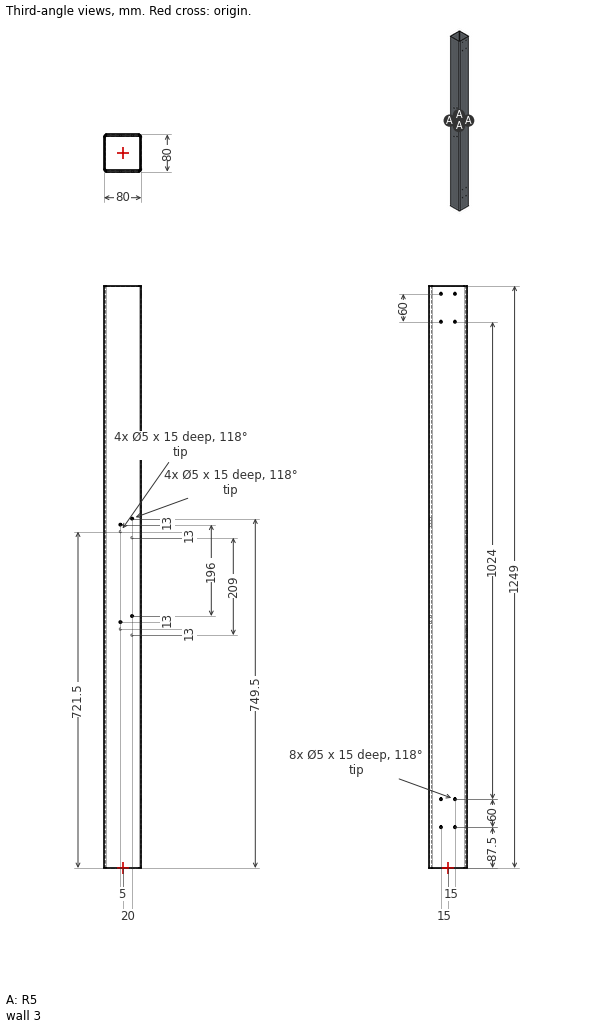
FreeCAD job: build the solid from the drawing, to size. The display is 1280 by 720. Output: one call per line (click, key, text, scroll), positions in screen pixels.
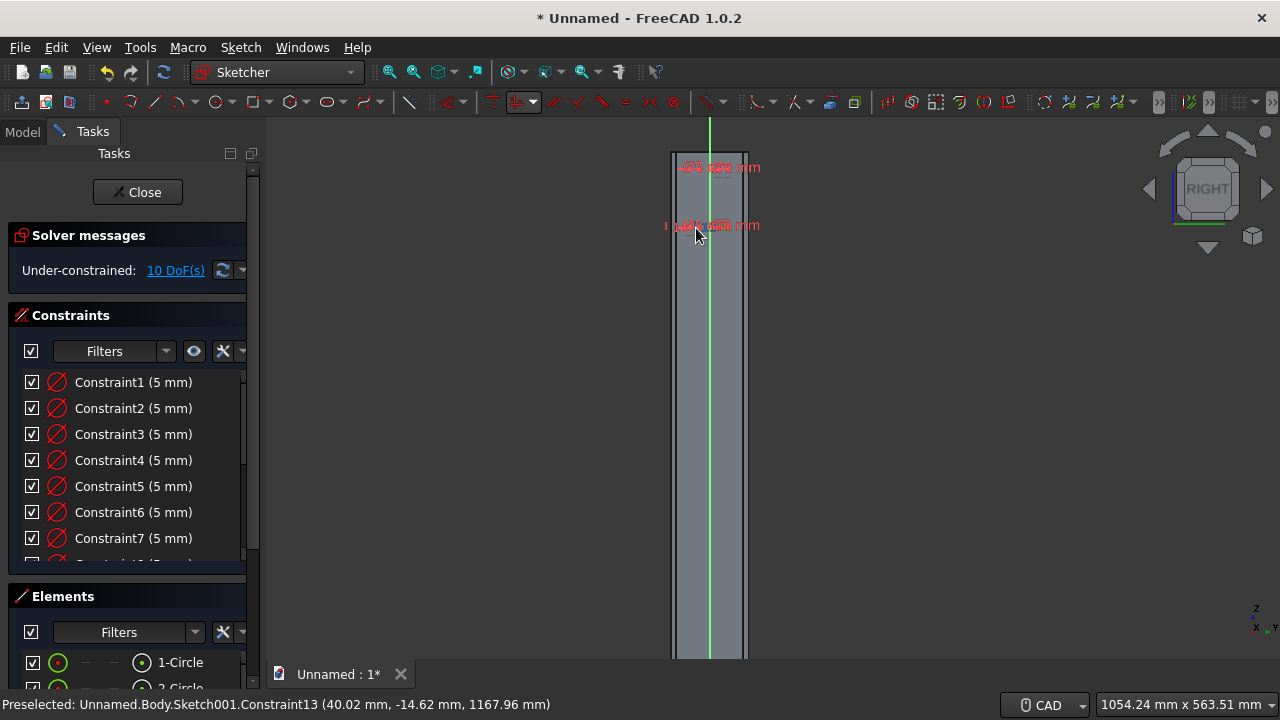
scroll(695, 228, up, 4)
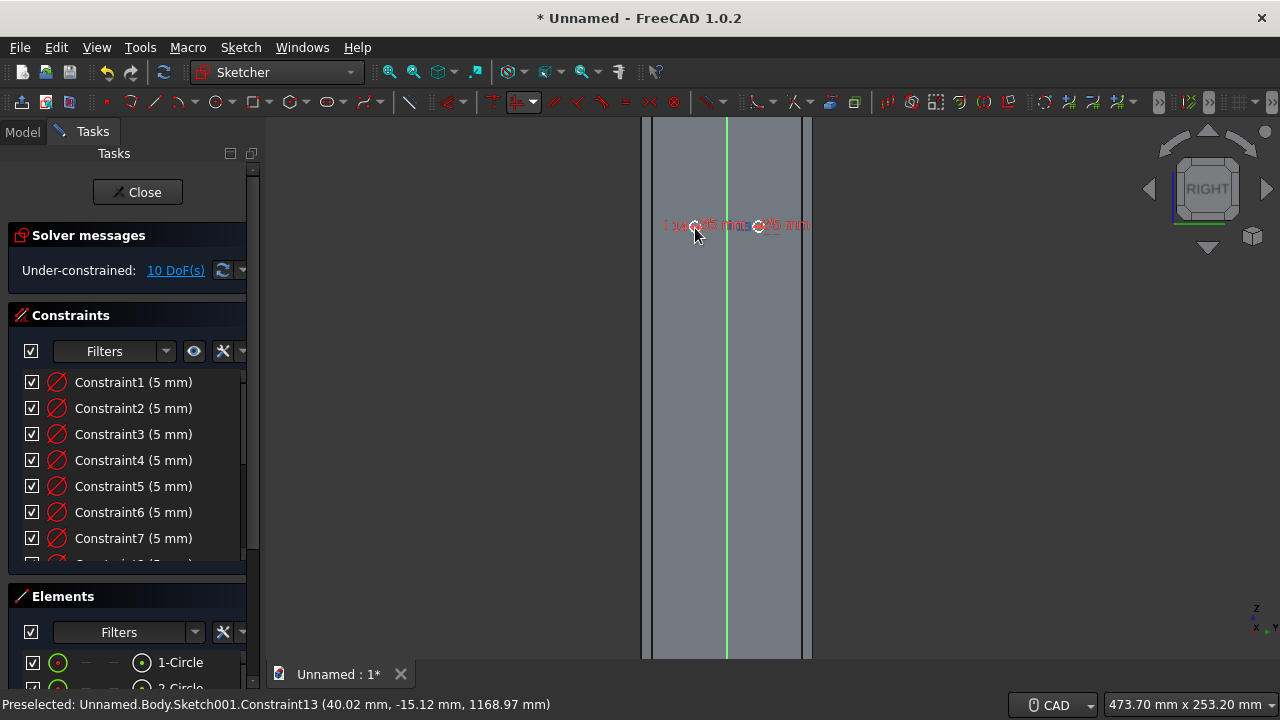
click(695, 227)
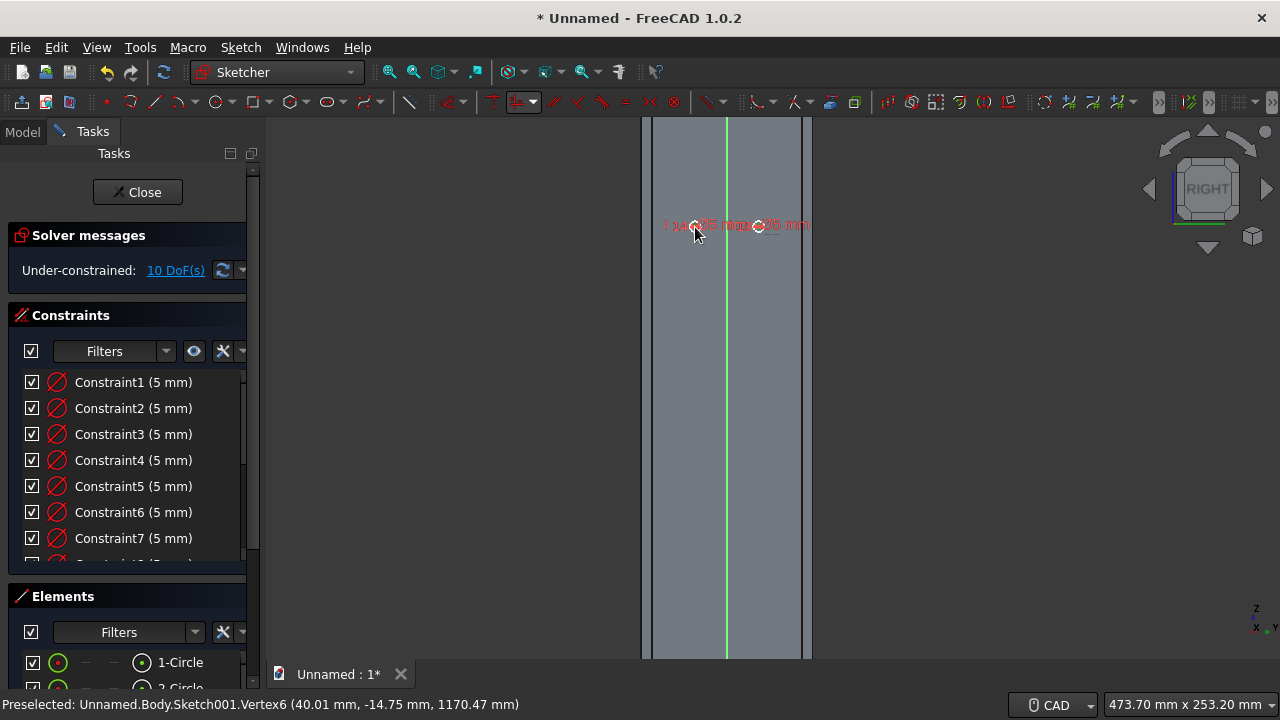
key(h)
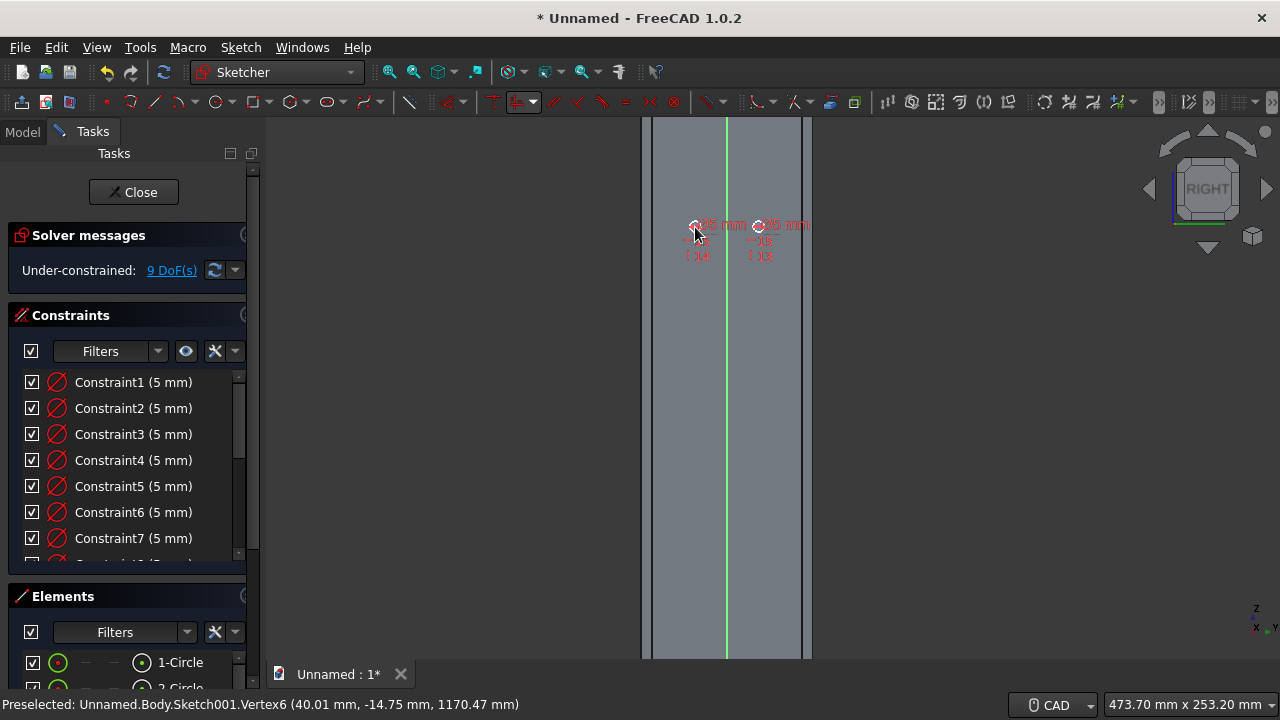
scroll(701, 228, down, 10)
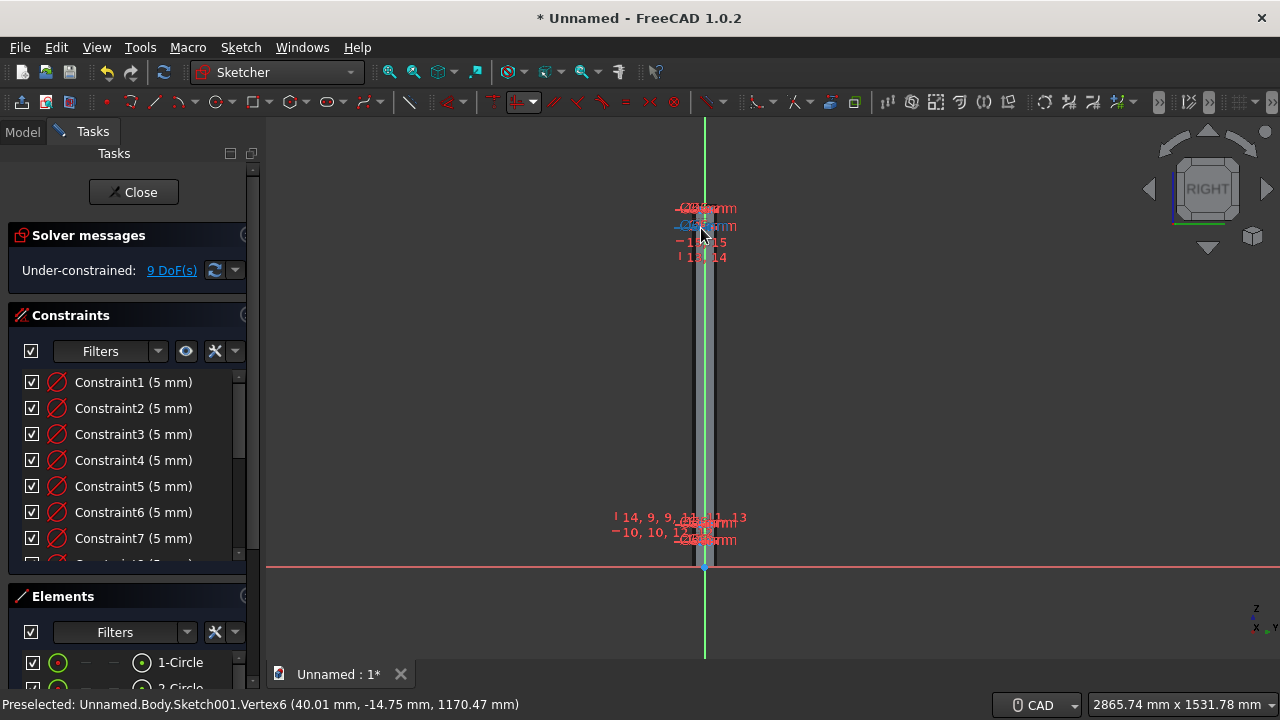
scroll(701, 228, up, 2)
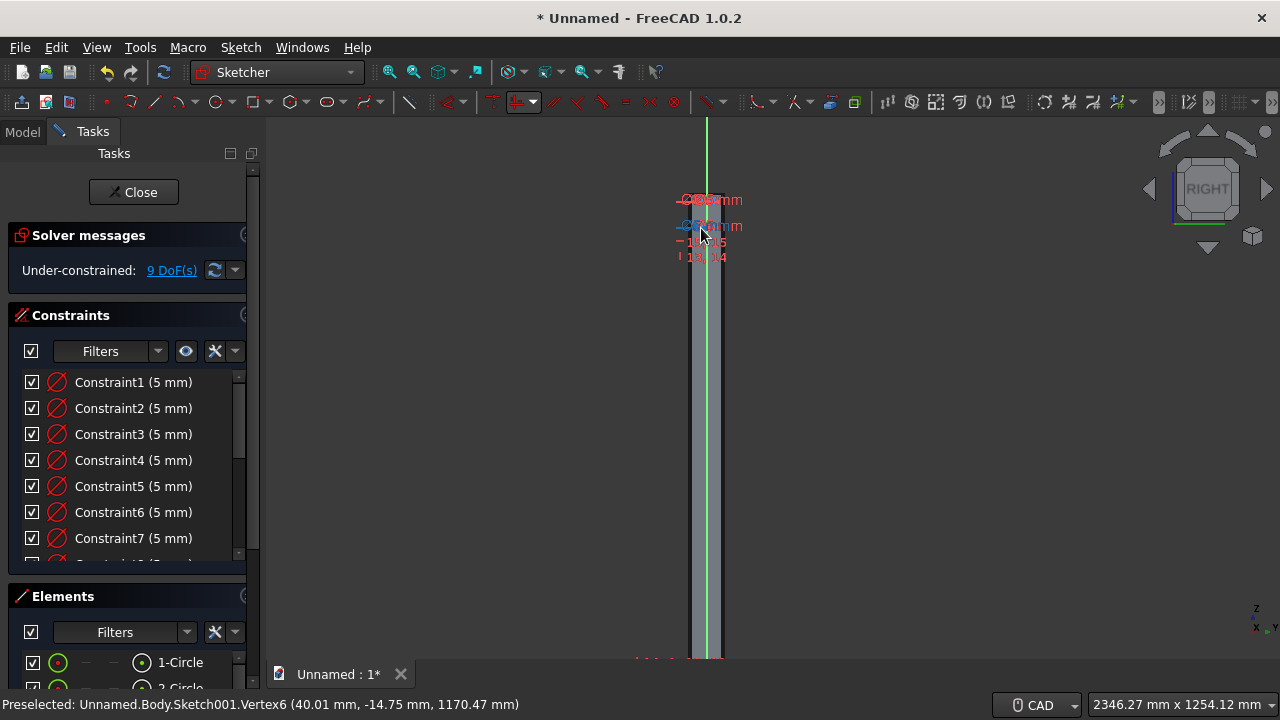
click(700, 228)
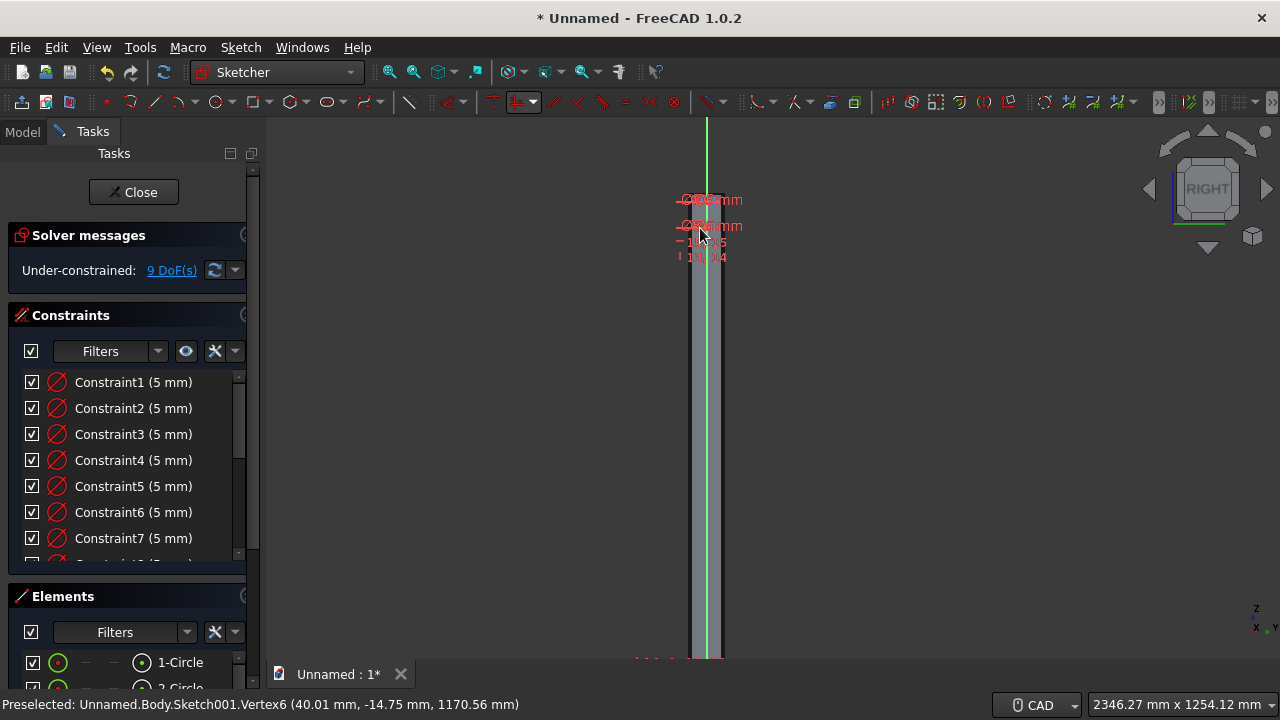
click(700, 202)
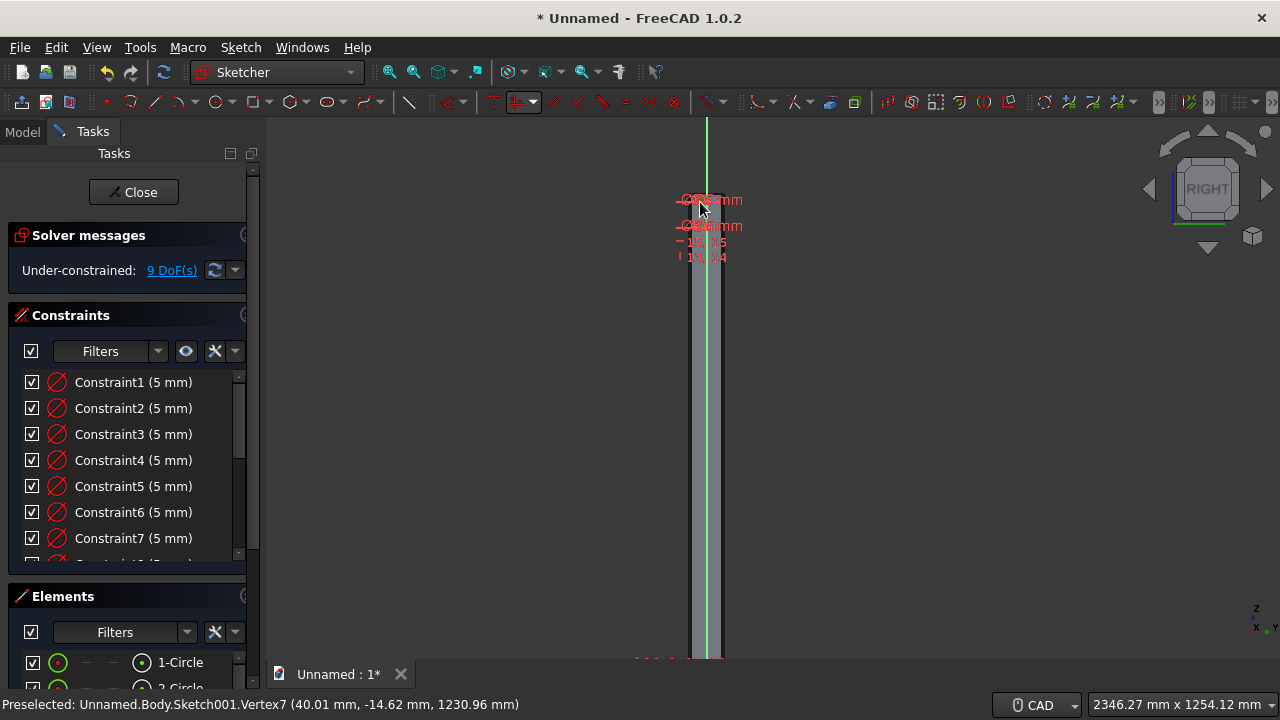
key(v)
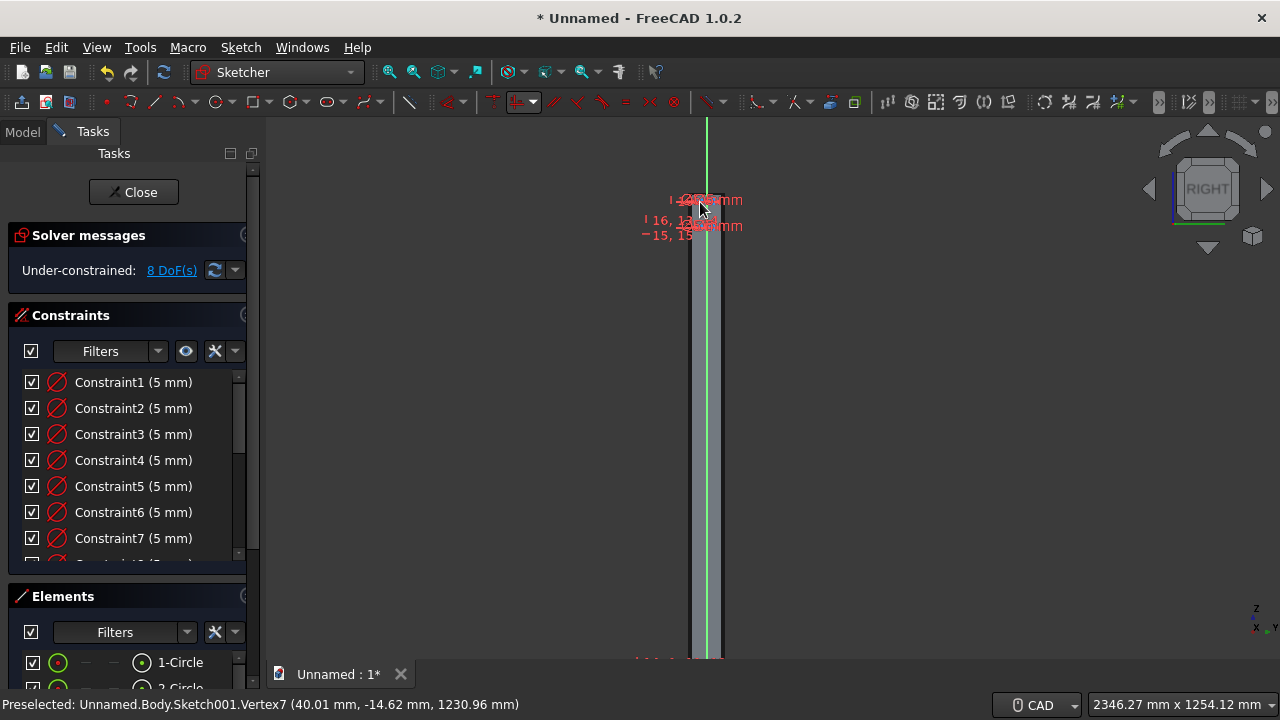
click(713, 228)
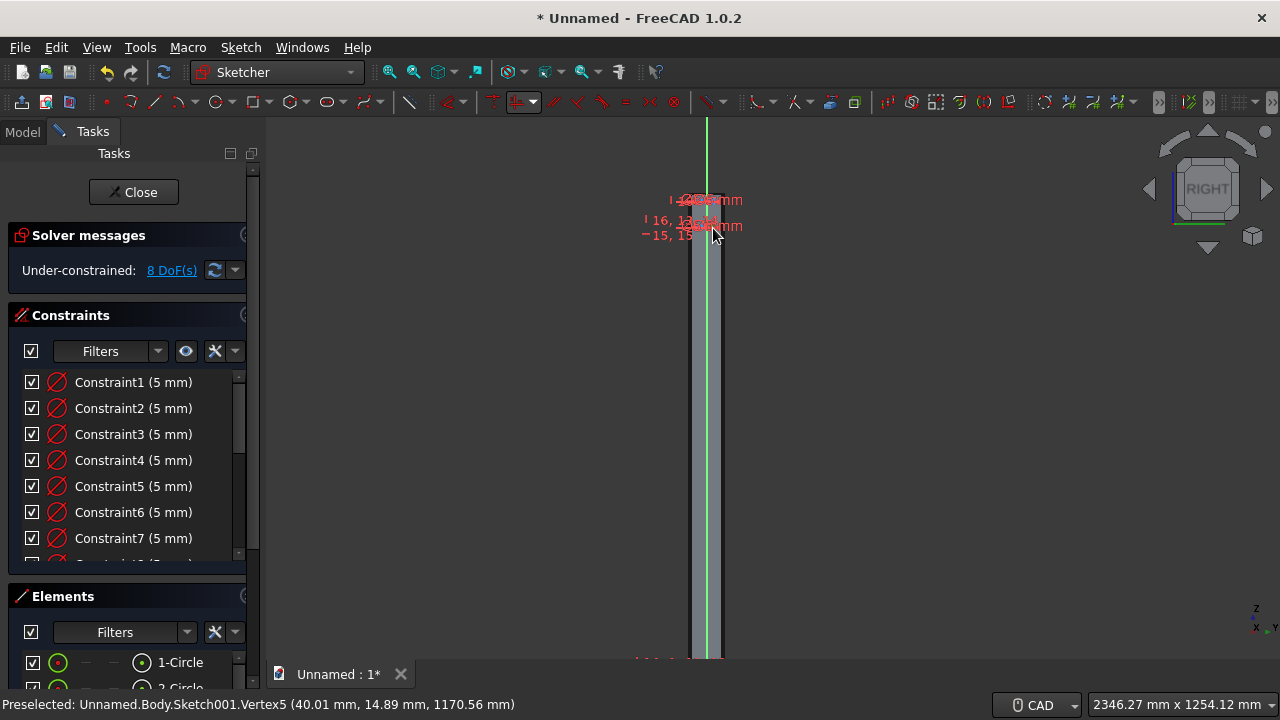
click(713, 202)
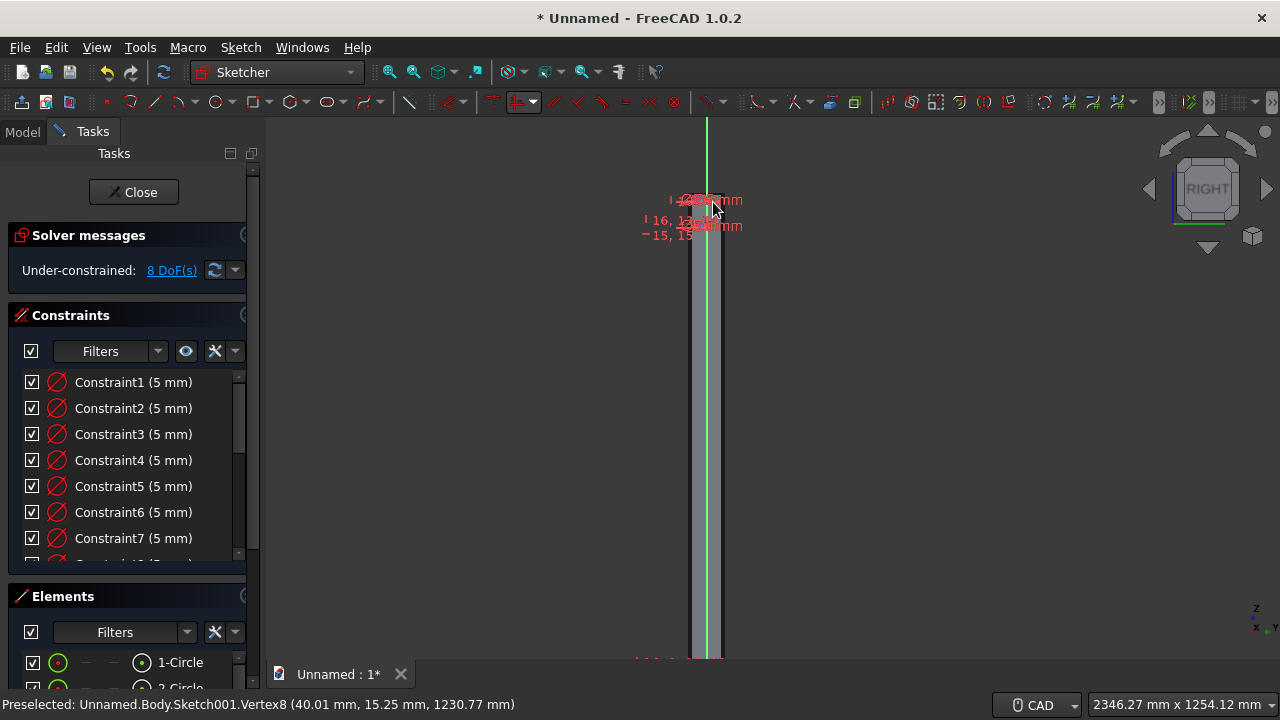
key(v)